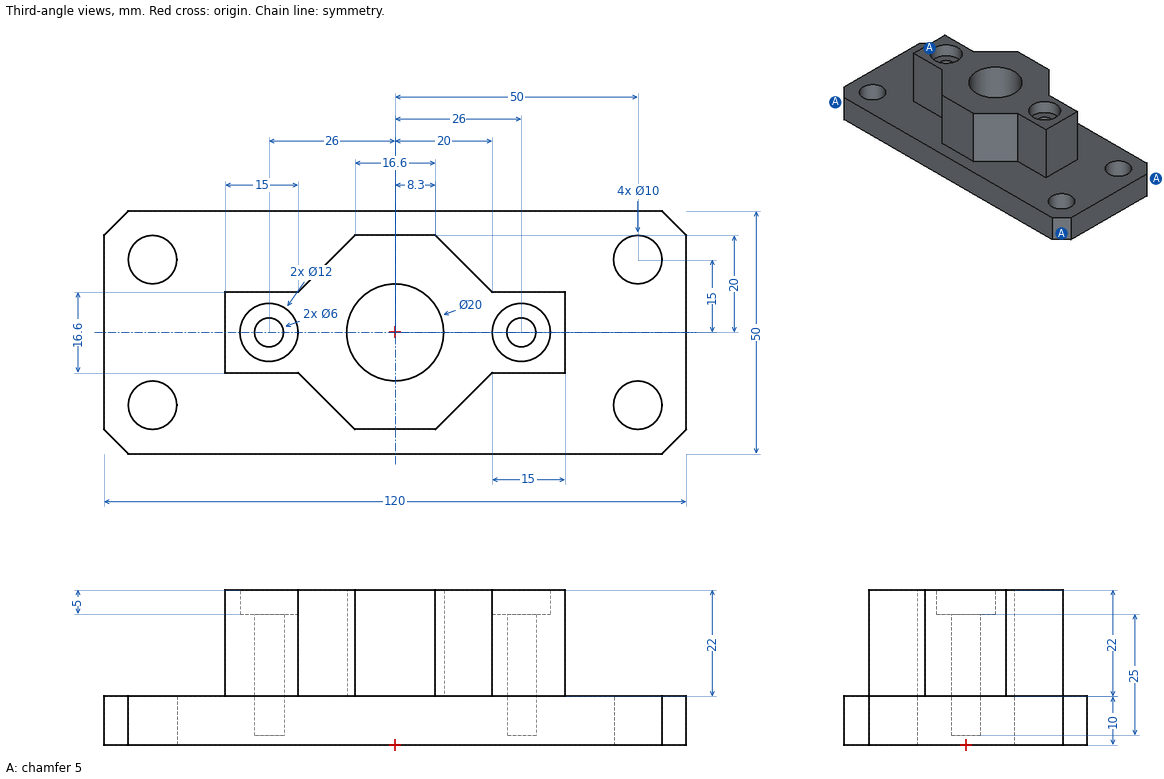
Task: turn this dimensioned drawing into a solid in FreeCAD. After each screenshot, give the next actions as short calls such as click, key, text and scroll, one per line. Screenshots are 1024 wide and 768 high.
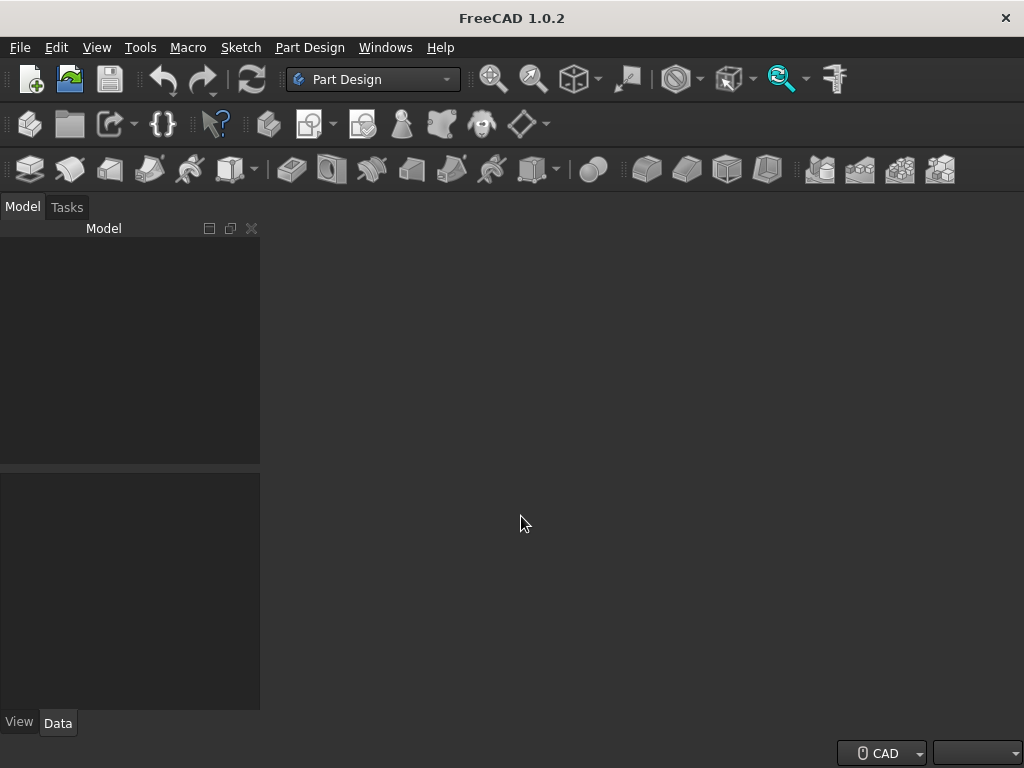
key(ctrl+n)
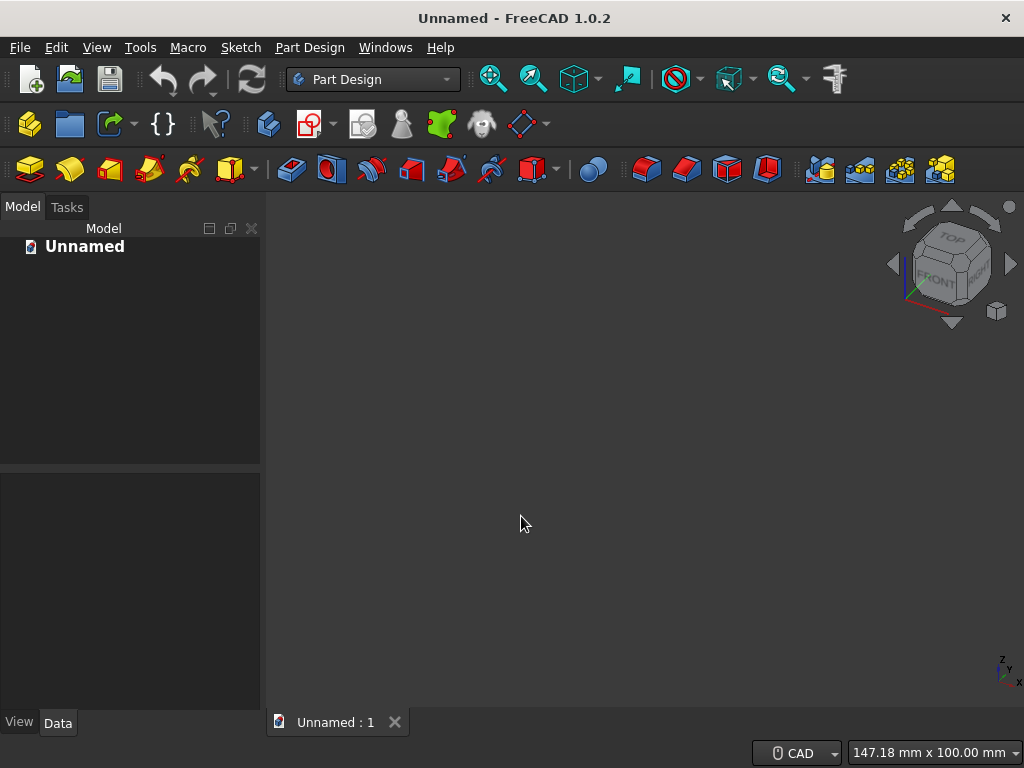
click(310, 124)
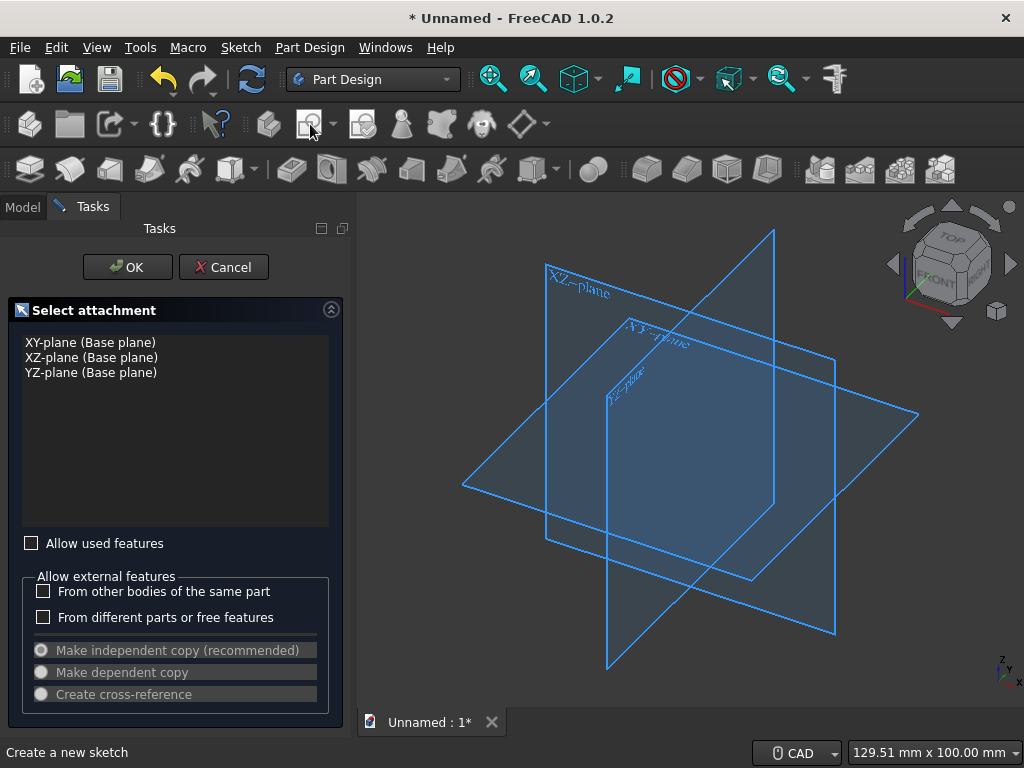
click(82, 342)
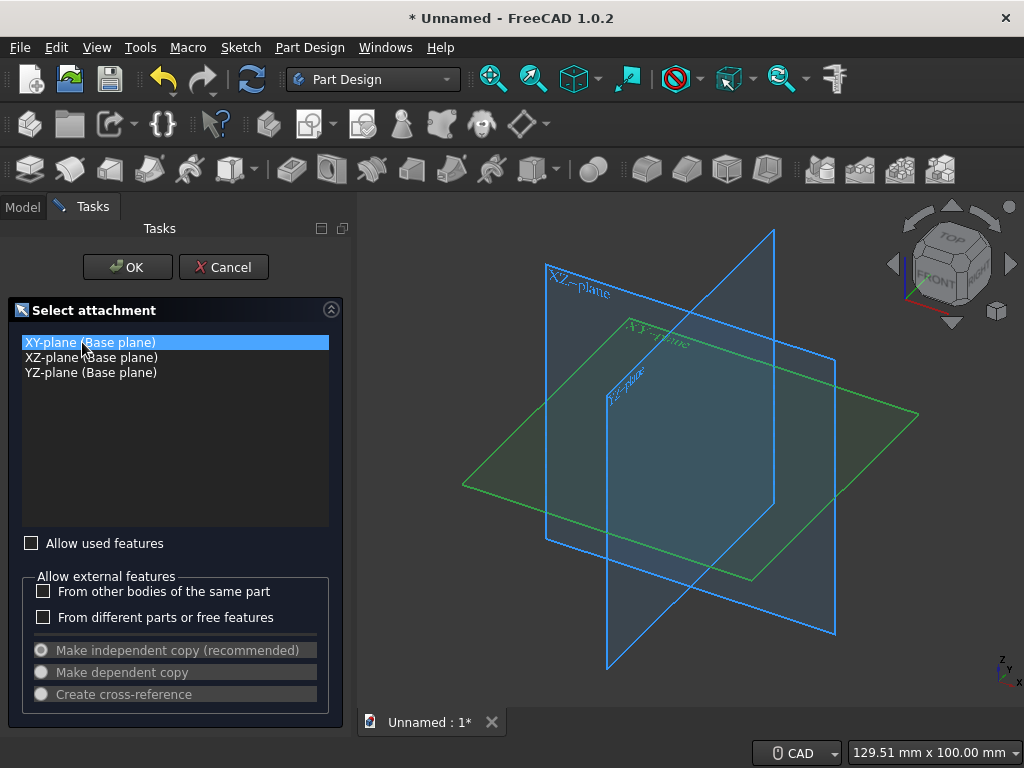
click(128, 267)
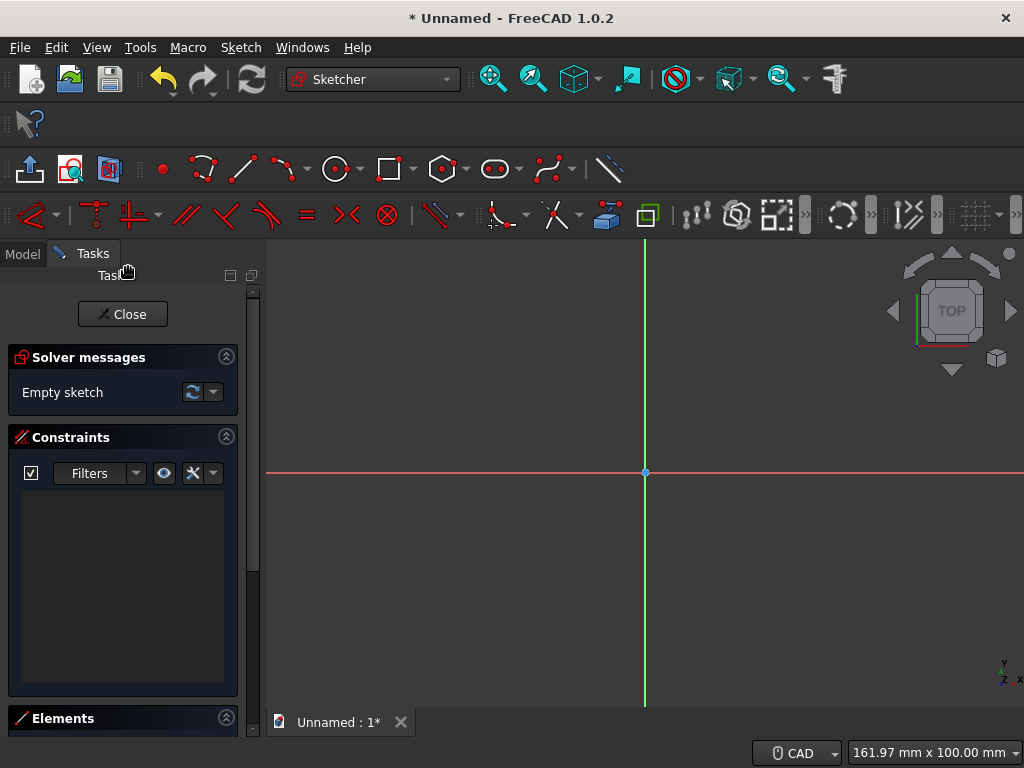
scroll(437, 473, down, 2)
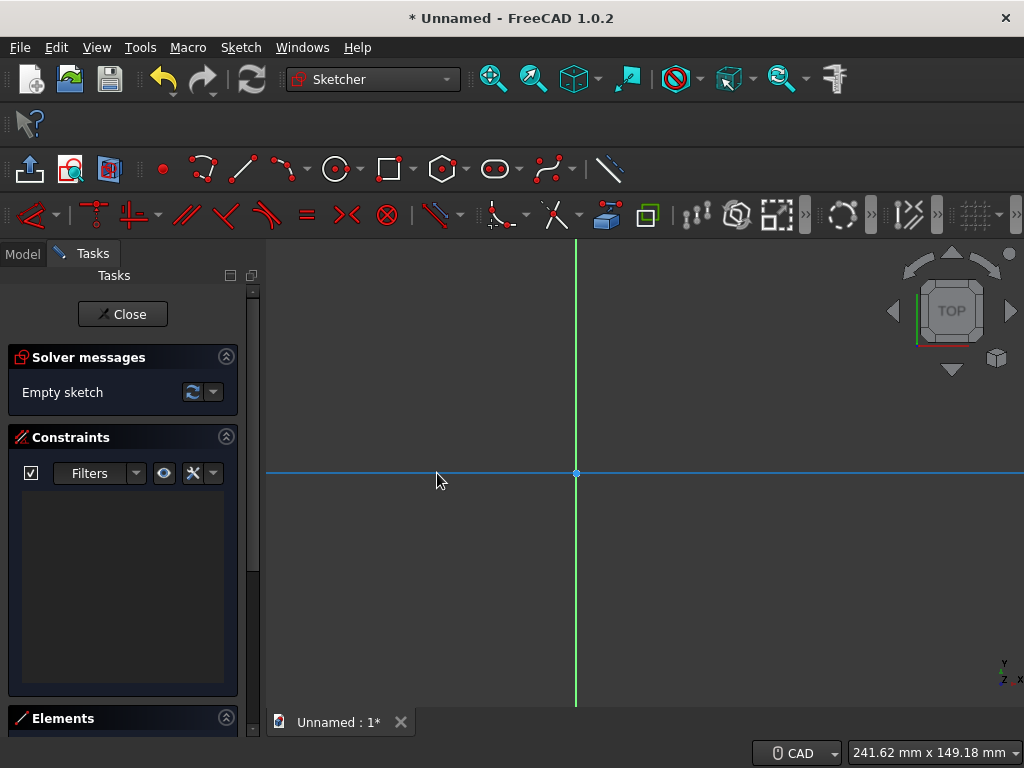
key(g)
key(v)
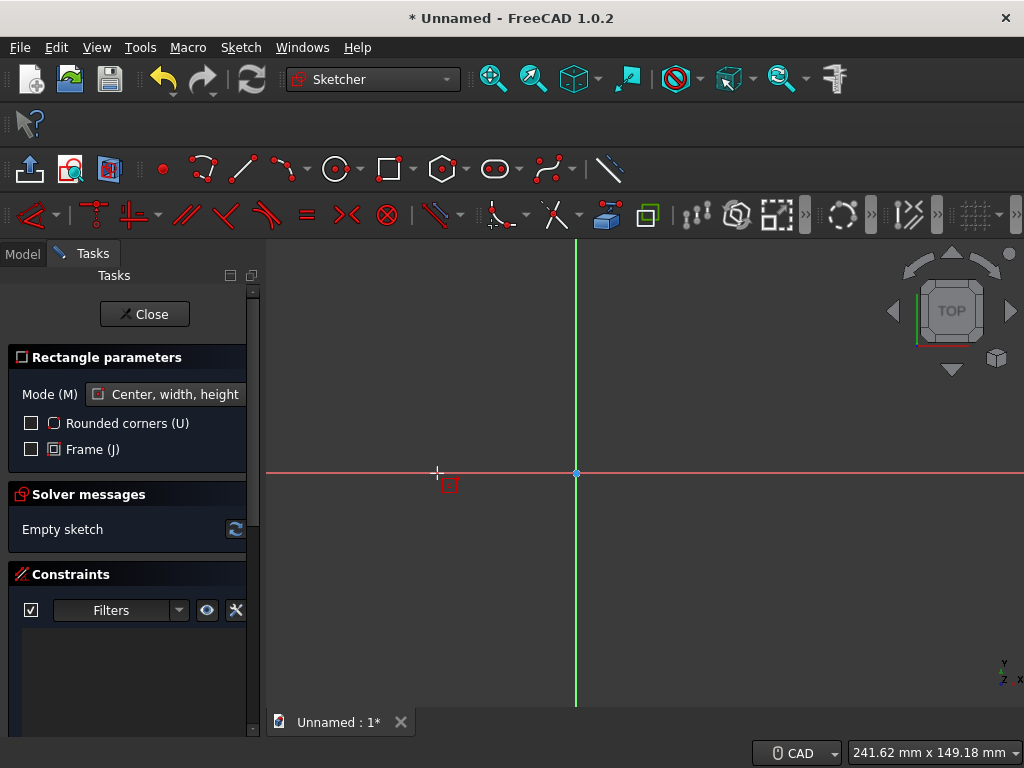
click(577, 473)
click(765, 395)
key(Escape)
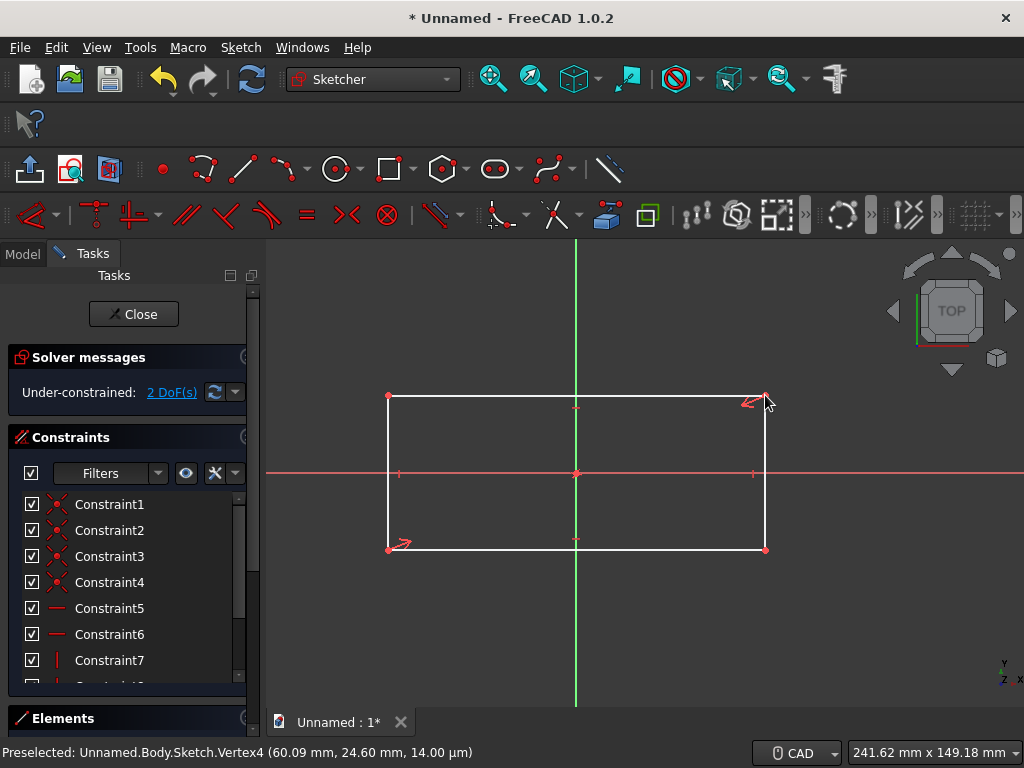
click(32, 216)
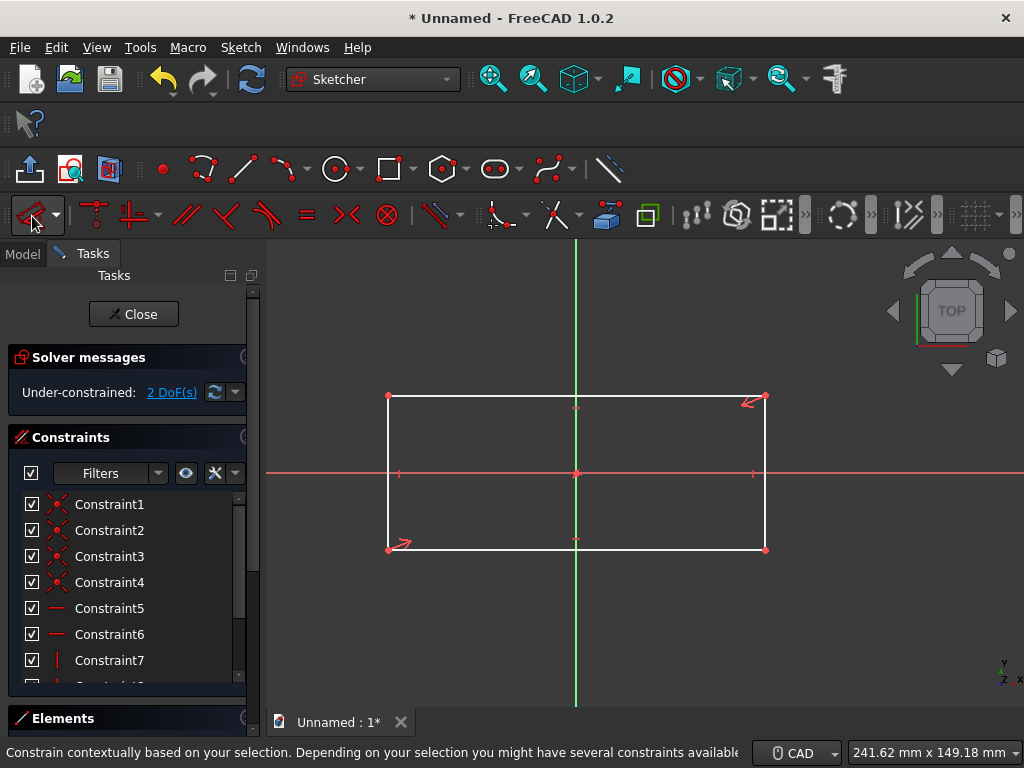
click(765, 504)
click(799, 438)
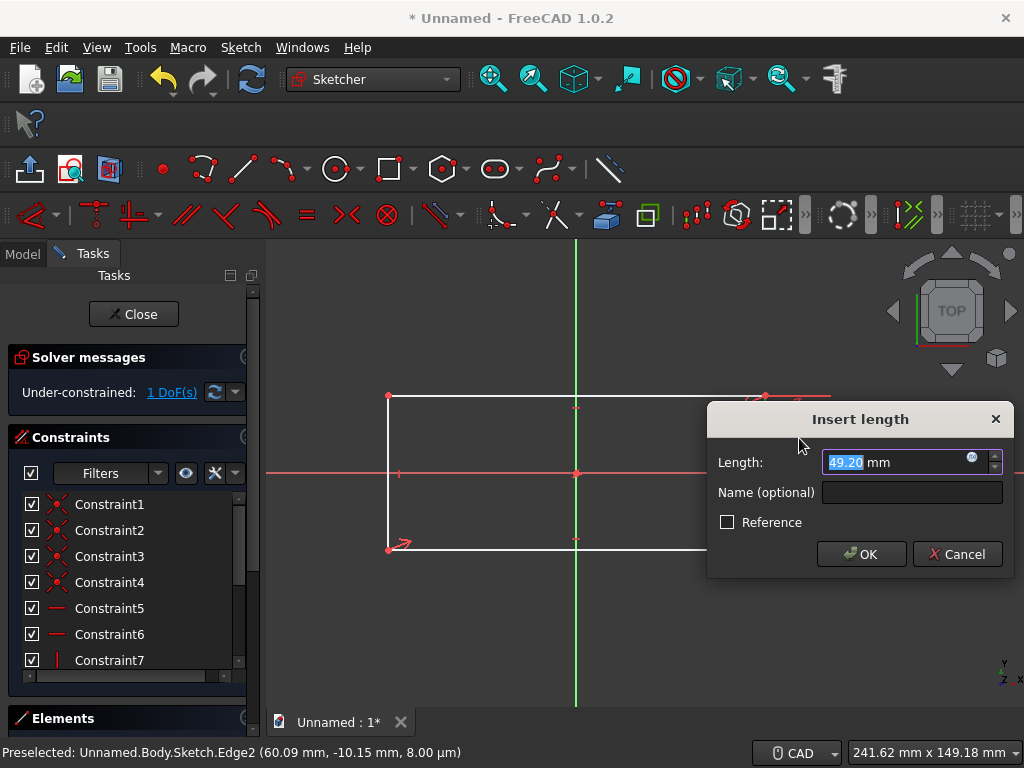
text(50)
key(Return)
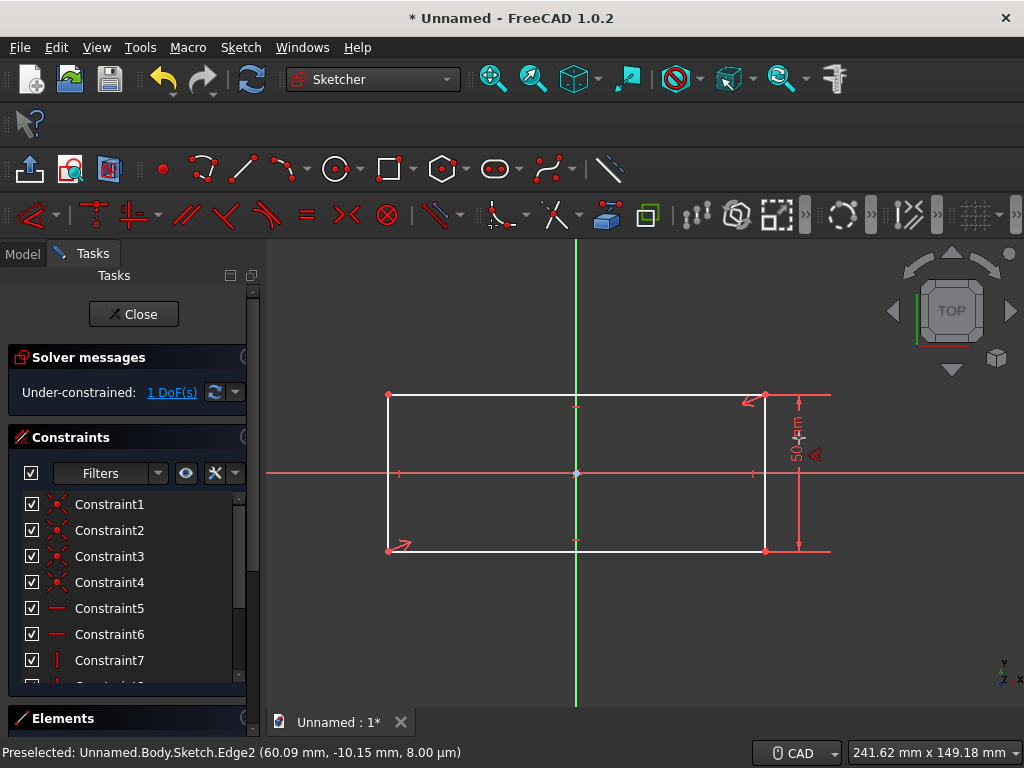
click(501, 552)
click(490, 586)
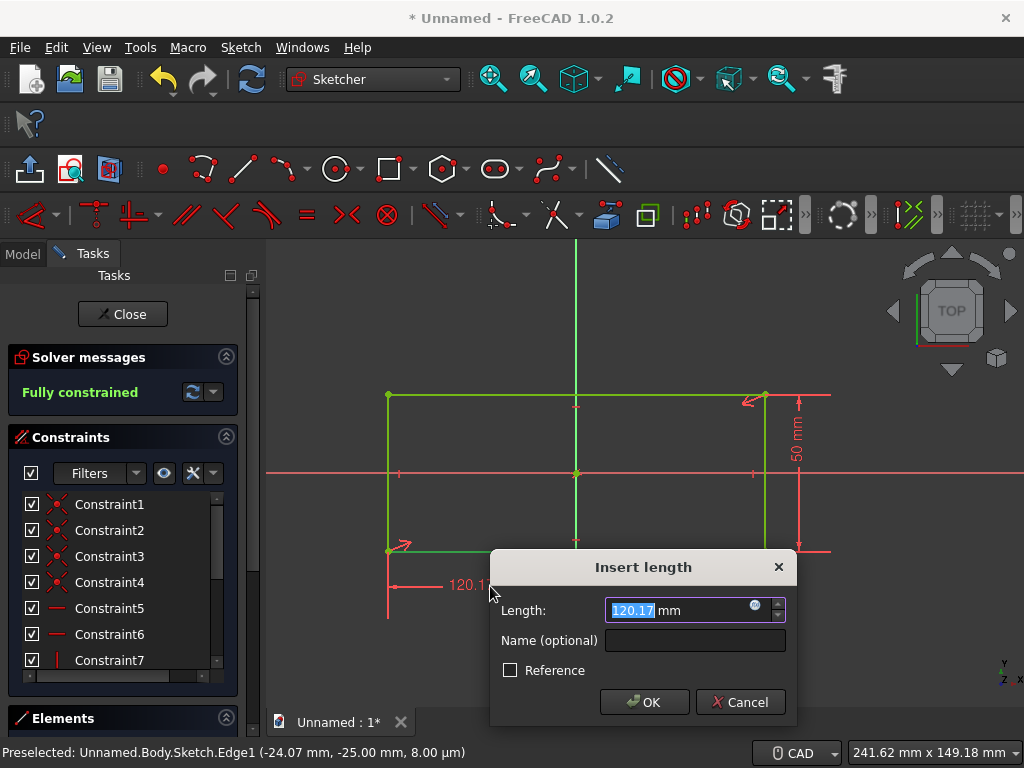
text(120)
key(Return)
key(Escape)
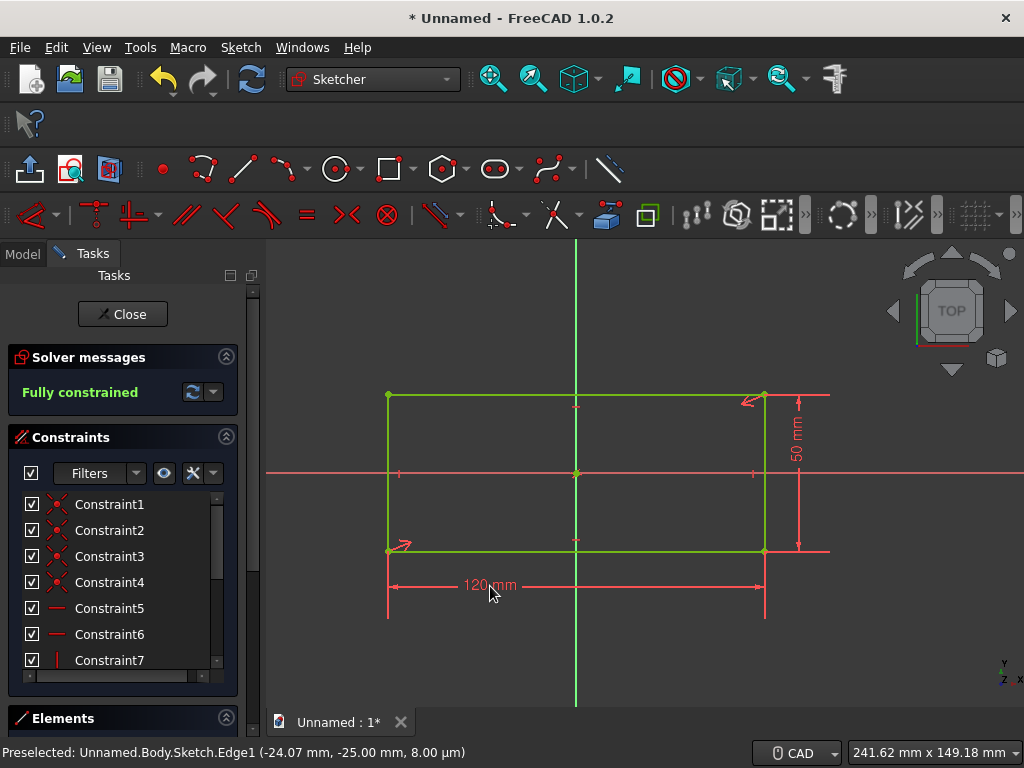
click(123, 314)